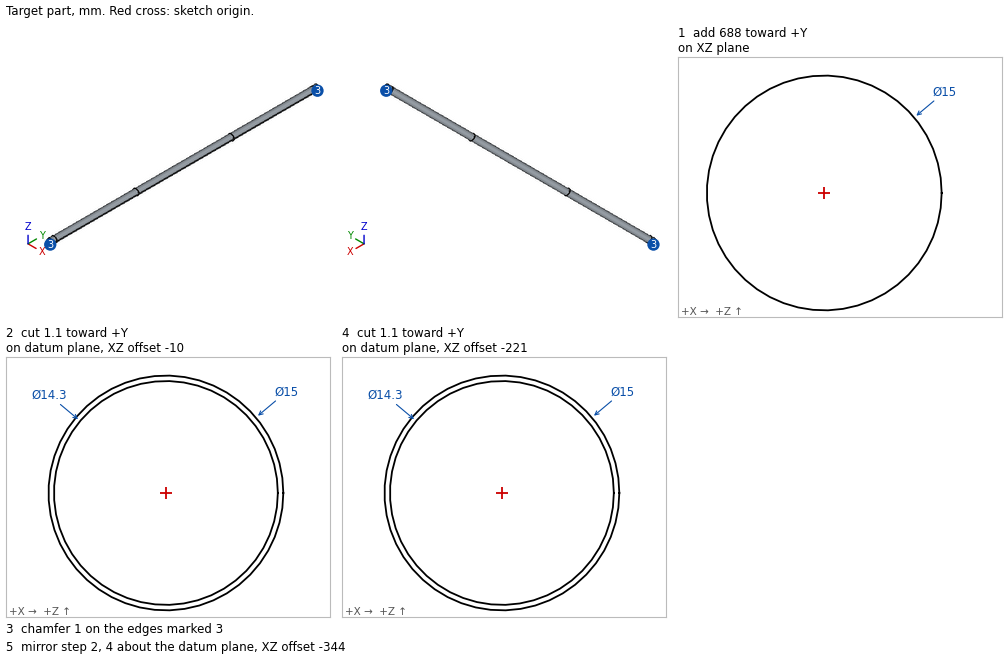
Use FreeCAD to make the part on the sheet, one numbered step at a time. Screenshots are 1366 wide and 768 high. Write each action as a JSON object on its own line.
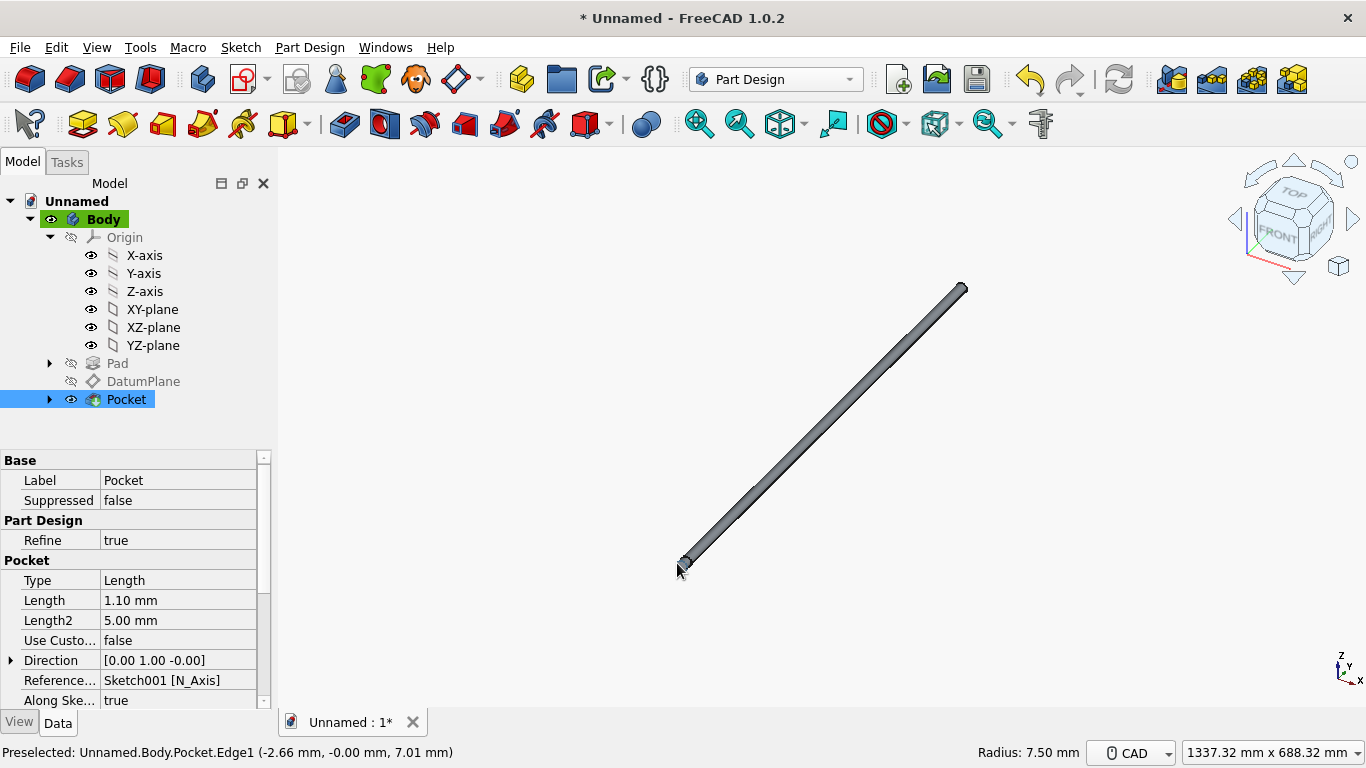
{"action": "key", "text": "0"}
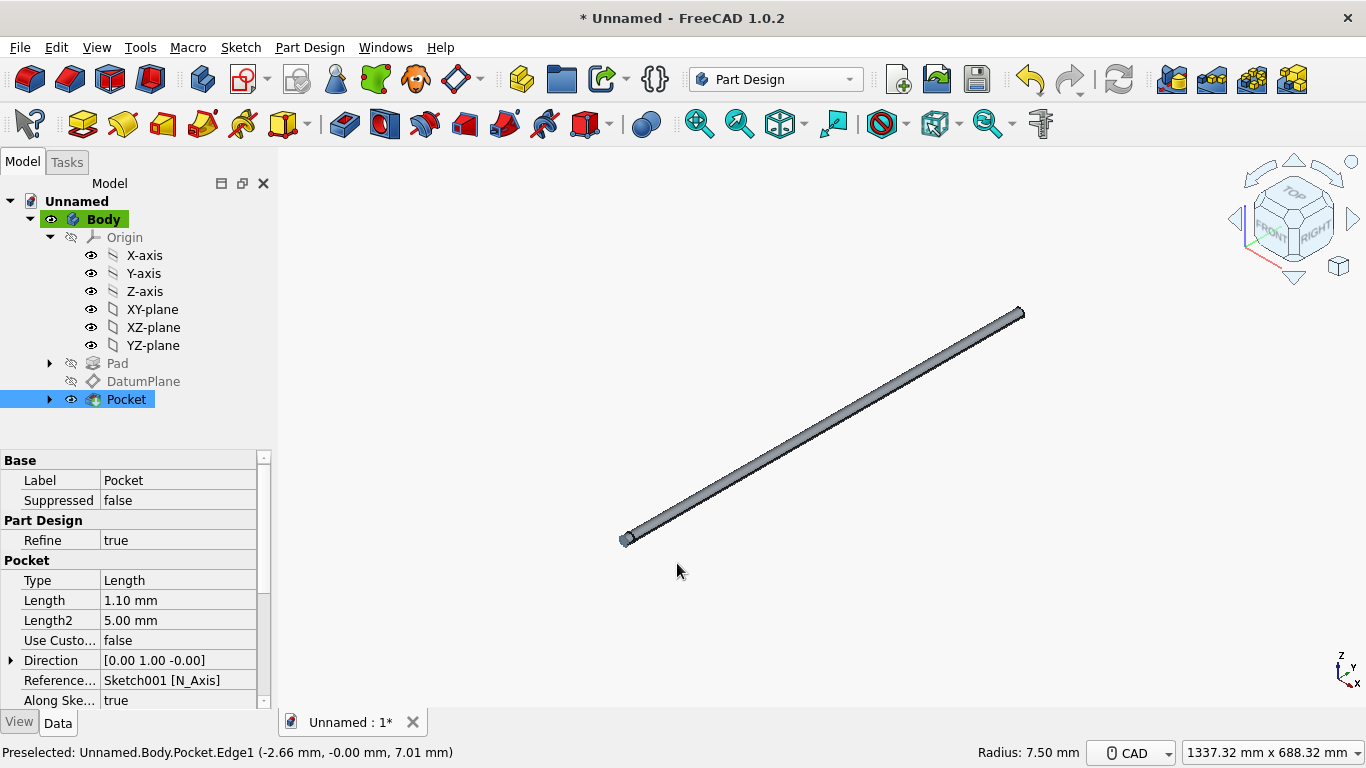
{"action": "left_click", "coordinate": [700, 124]}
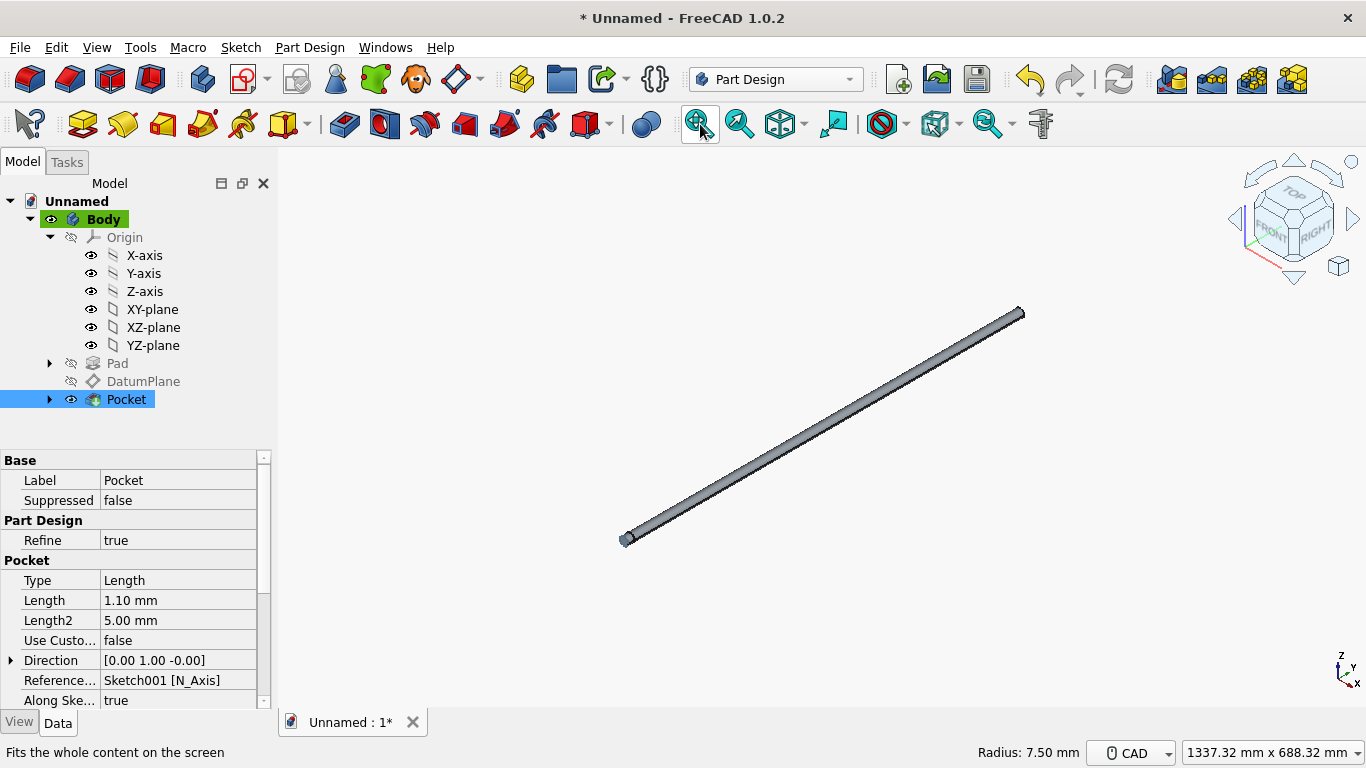
{"action": "left_click", "coordinate": [1019, 306], "text": "ctrl"}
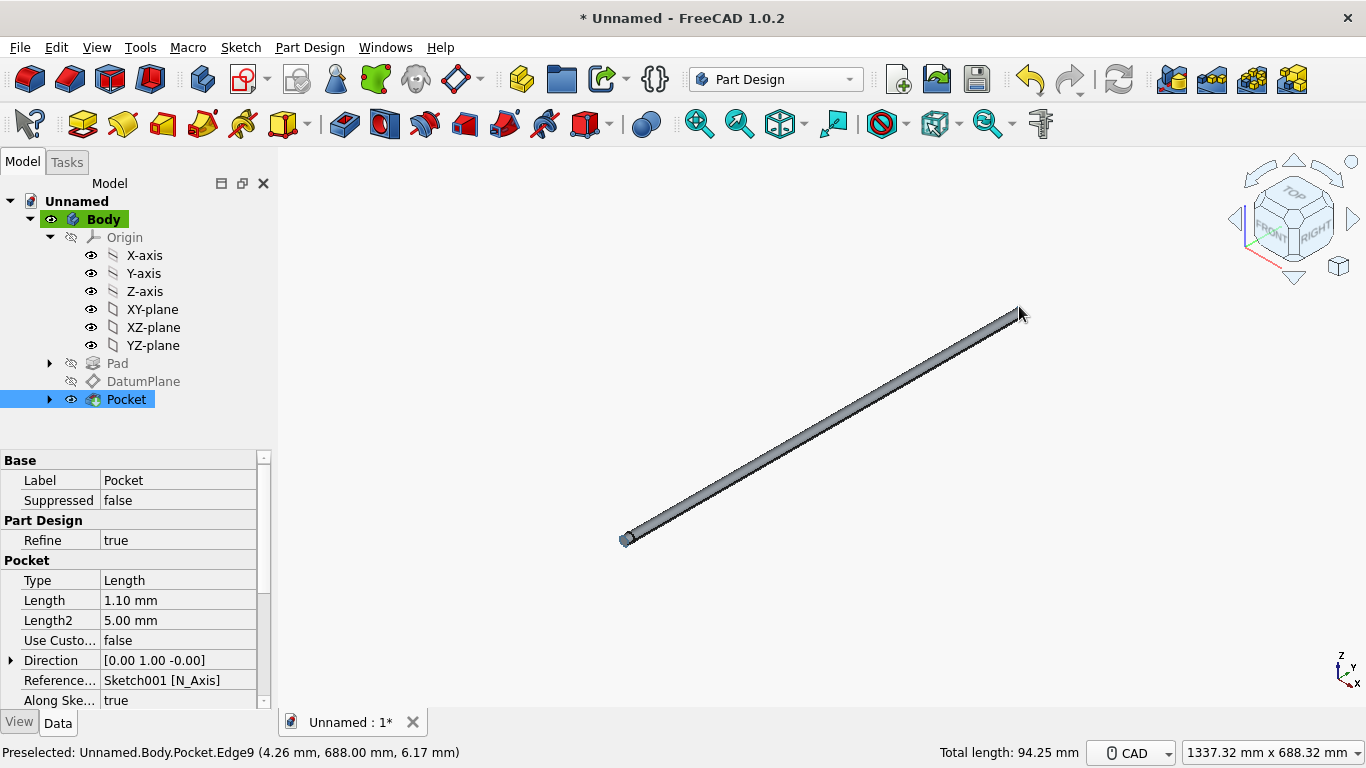
{"action": "left_click", "coordinate": [70, 80]}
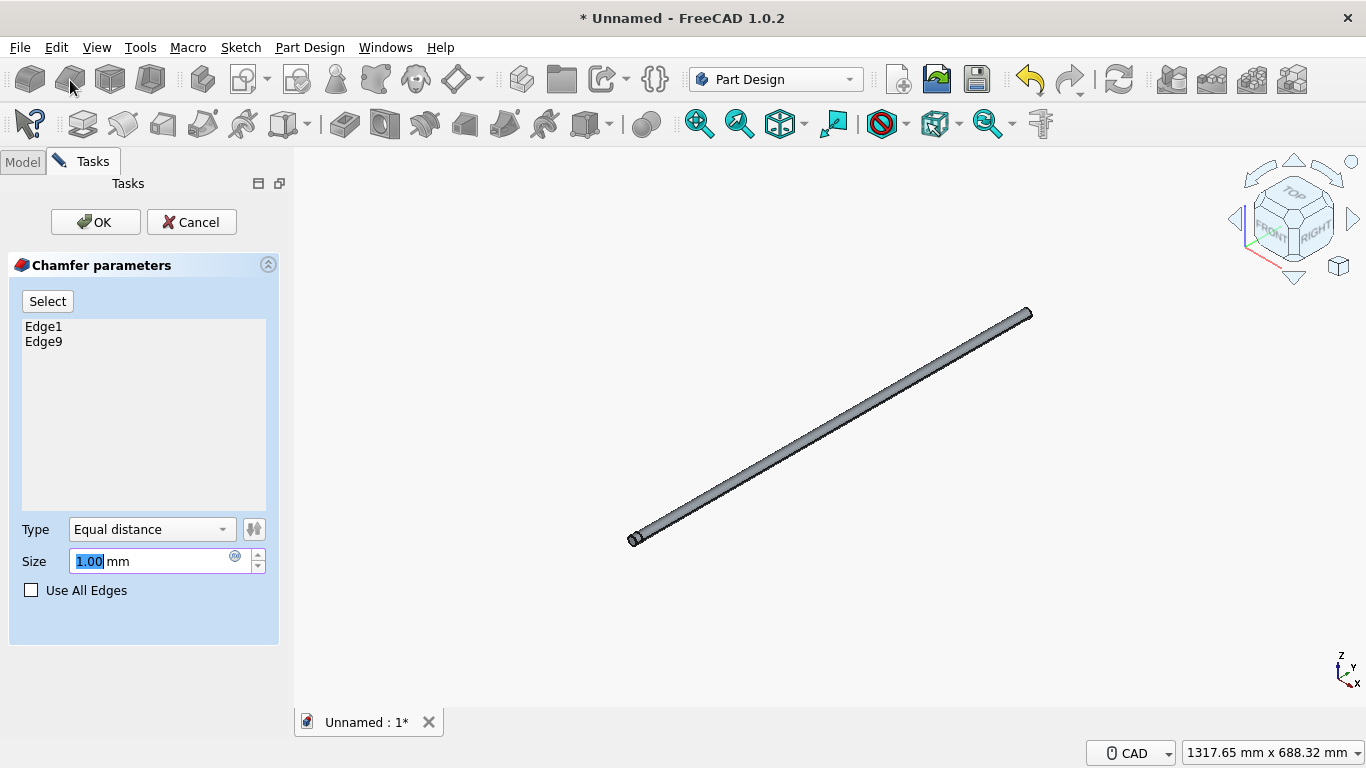
{"action": "type", "text": "1"}
{"action": "key", "text": "Tab"}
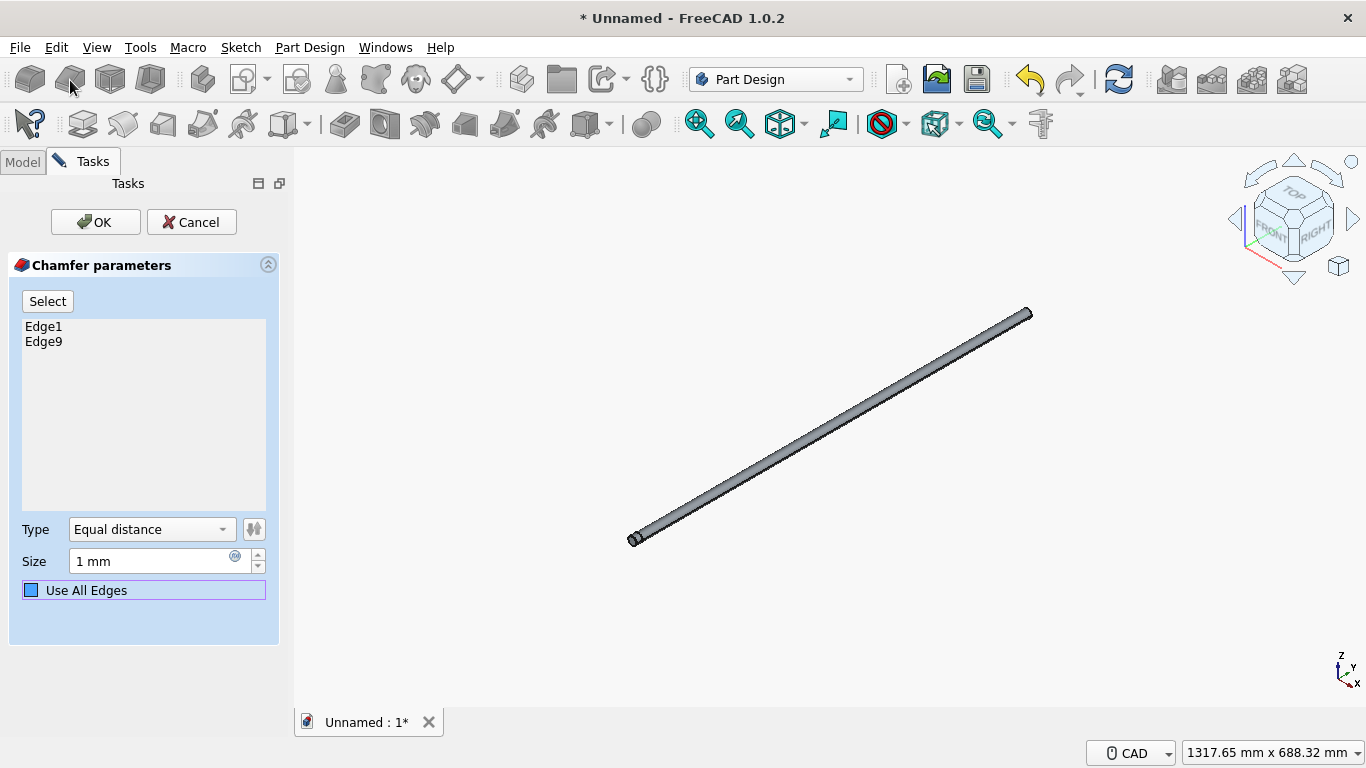
{"action": "left_click", "coordinate": [96, 222]}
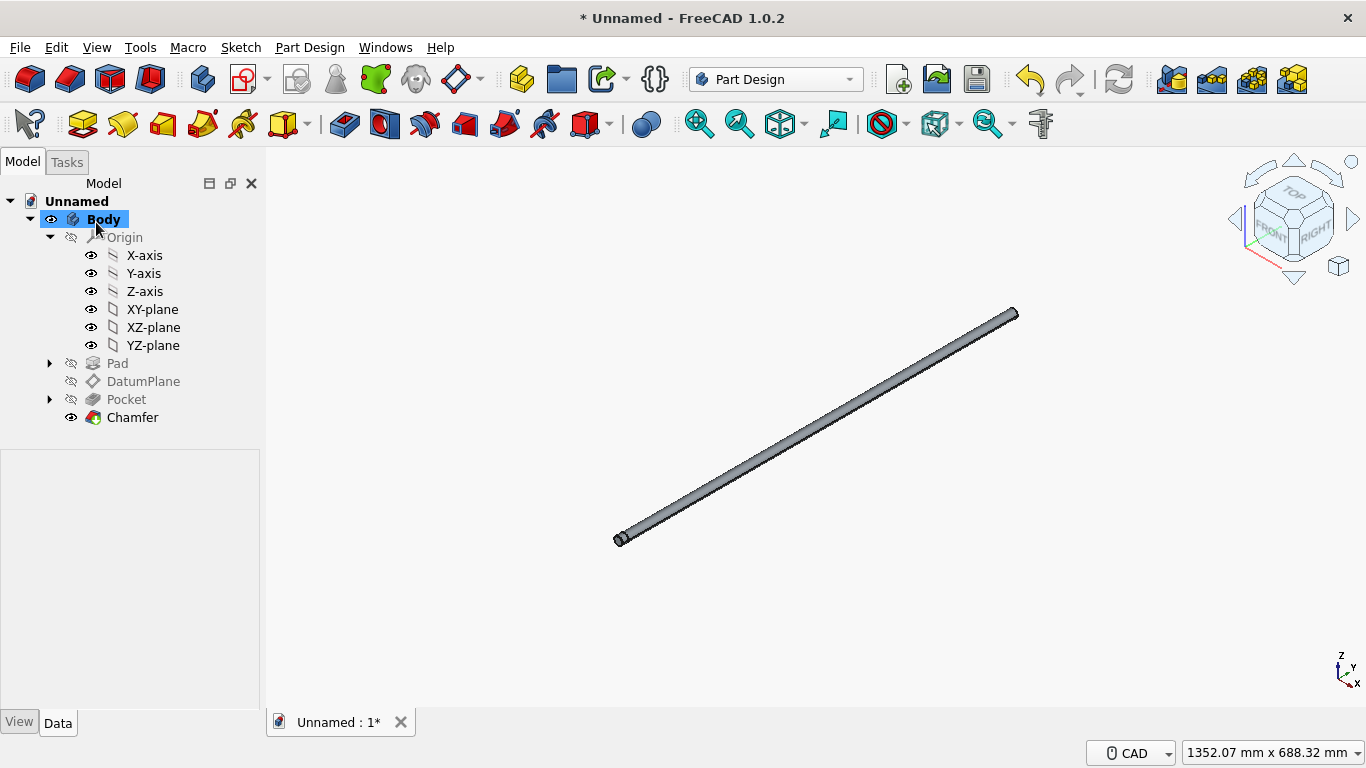
{"action": "left_click", "coordinate": [700, 124]}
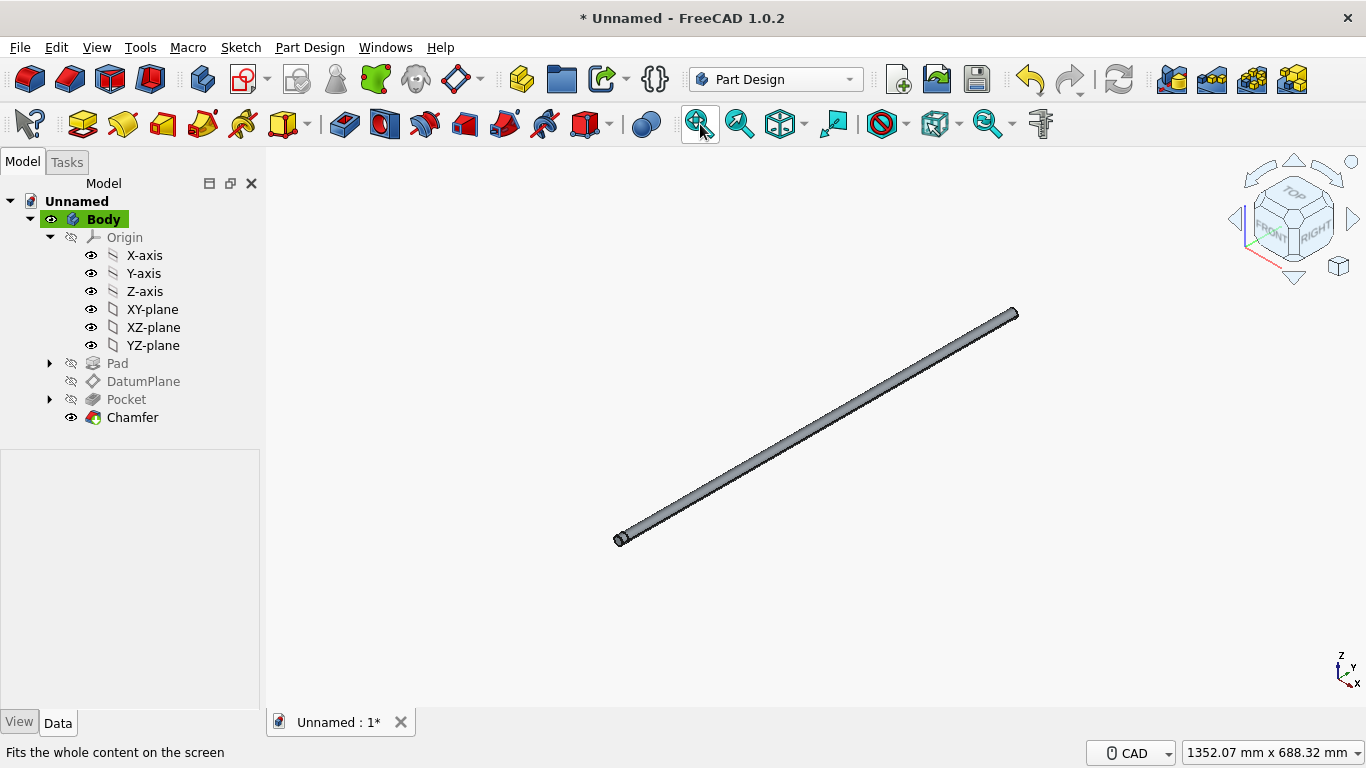
{"action": "left_click", "coordinate": [136, 327]}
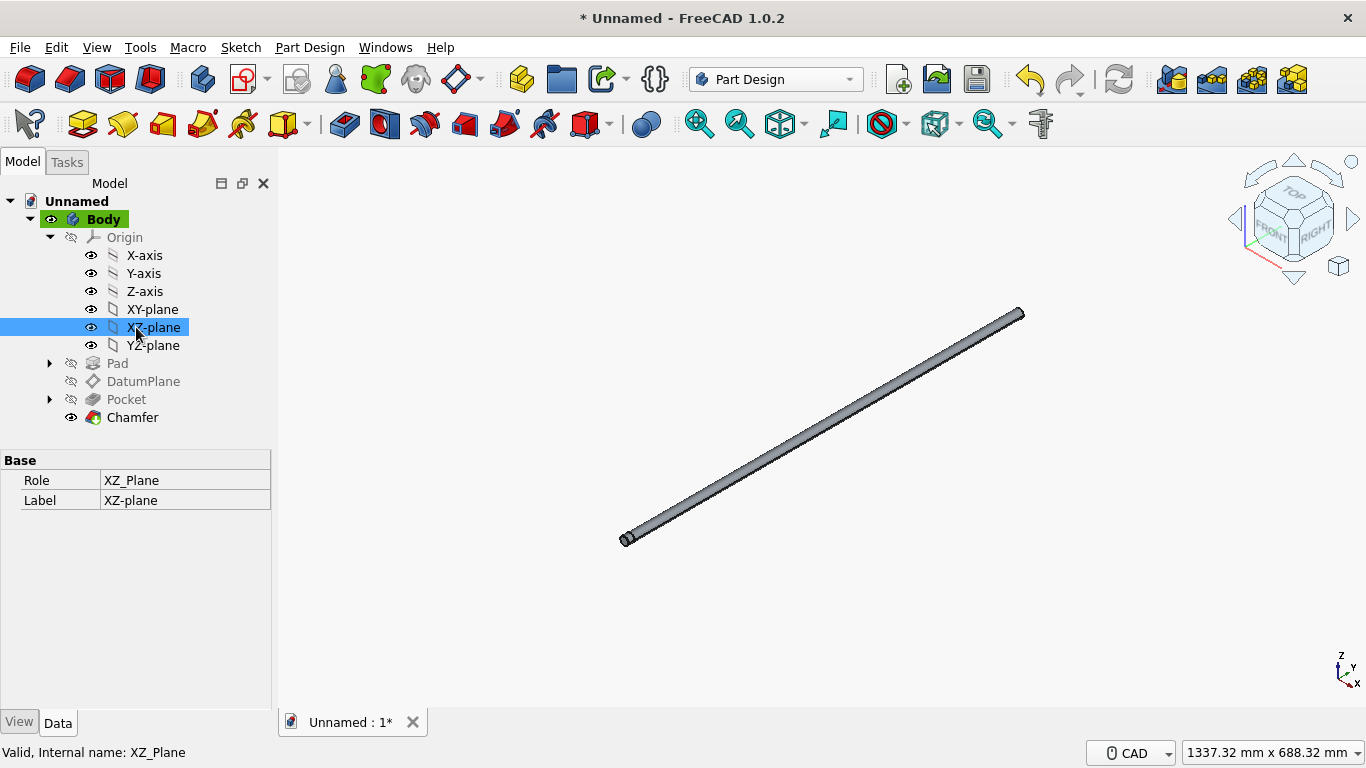
{"action": "left_click", "coordinate": [456, 80]}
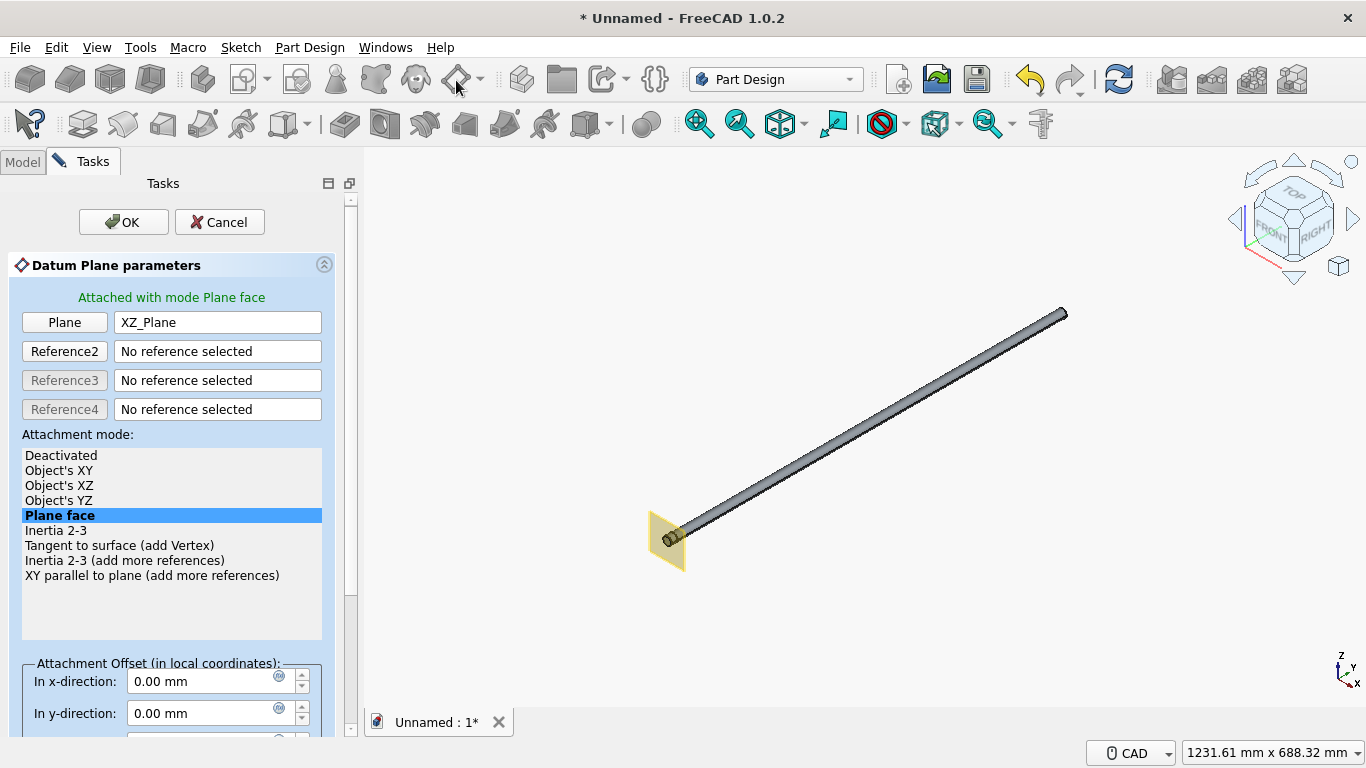
{"action": "scroll", "coordinate": [351, 464], "scroll_direction": "down", "scroll_amount": 2}